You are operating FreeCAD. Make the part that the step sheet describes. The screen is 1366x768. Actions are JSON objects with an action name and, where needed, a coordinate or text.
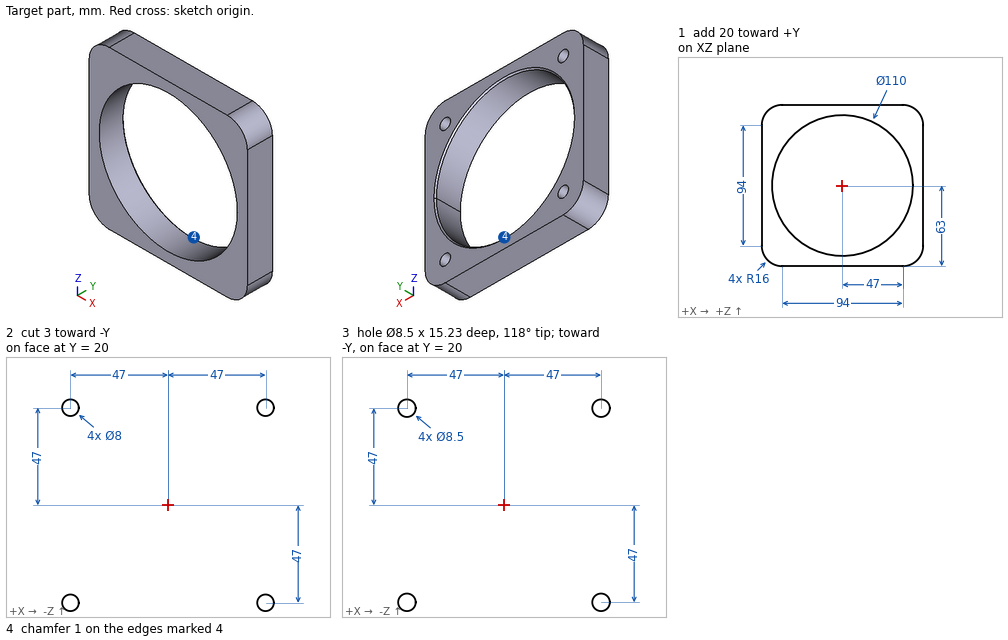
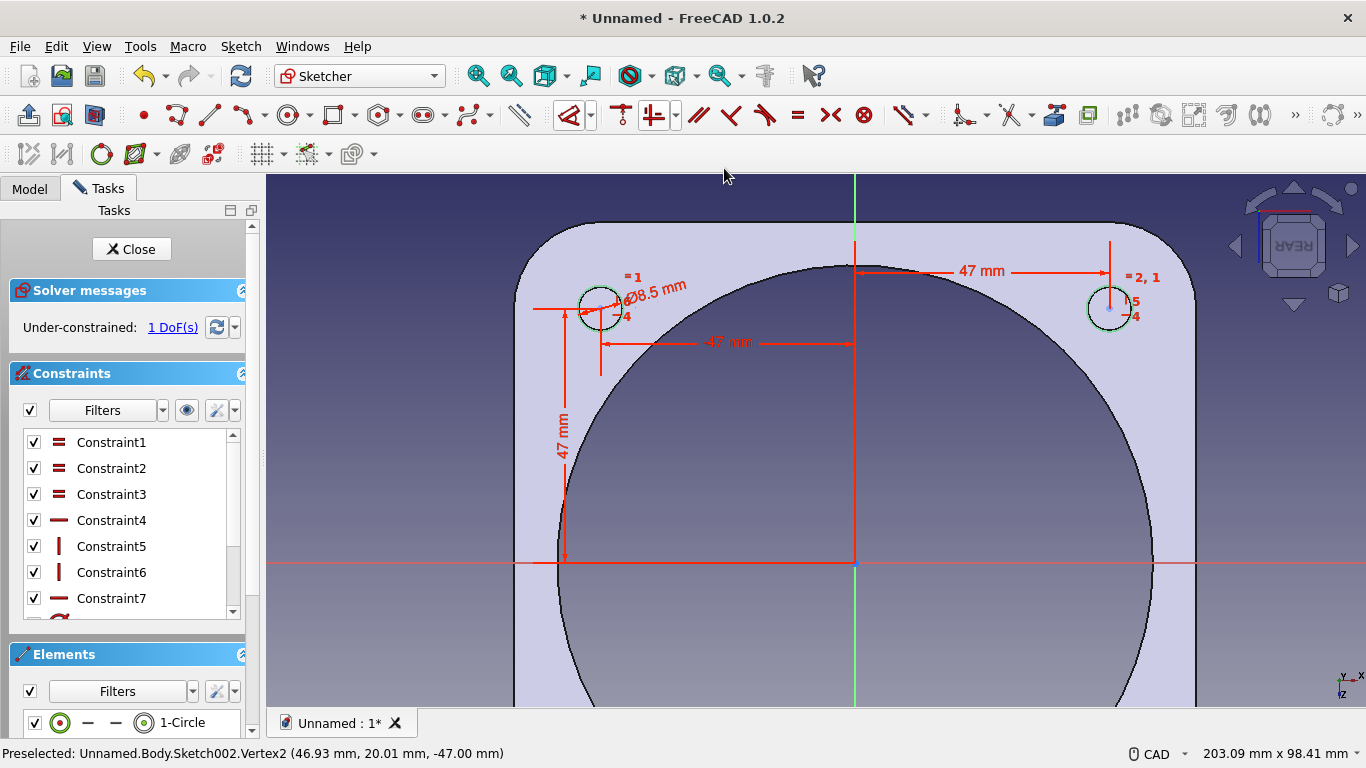
{"action": "scroll", "coordinate": [617, 291], "scroll_direction": "down", "scroll_amount": 3}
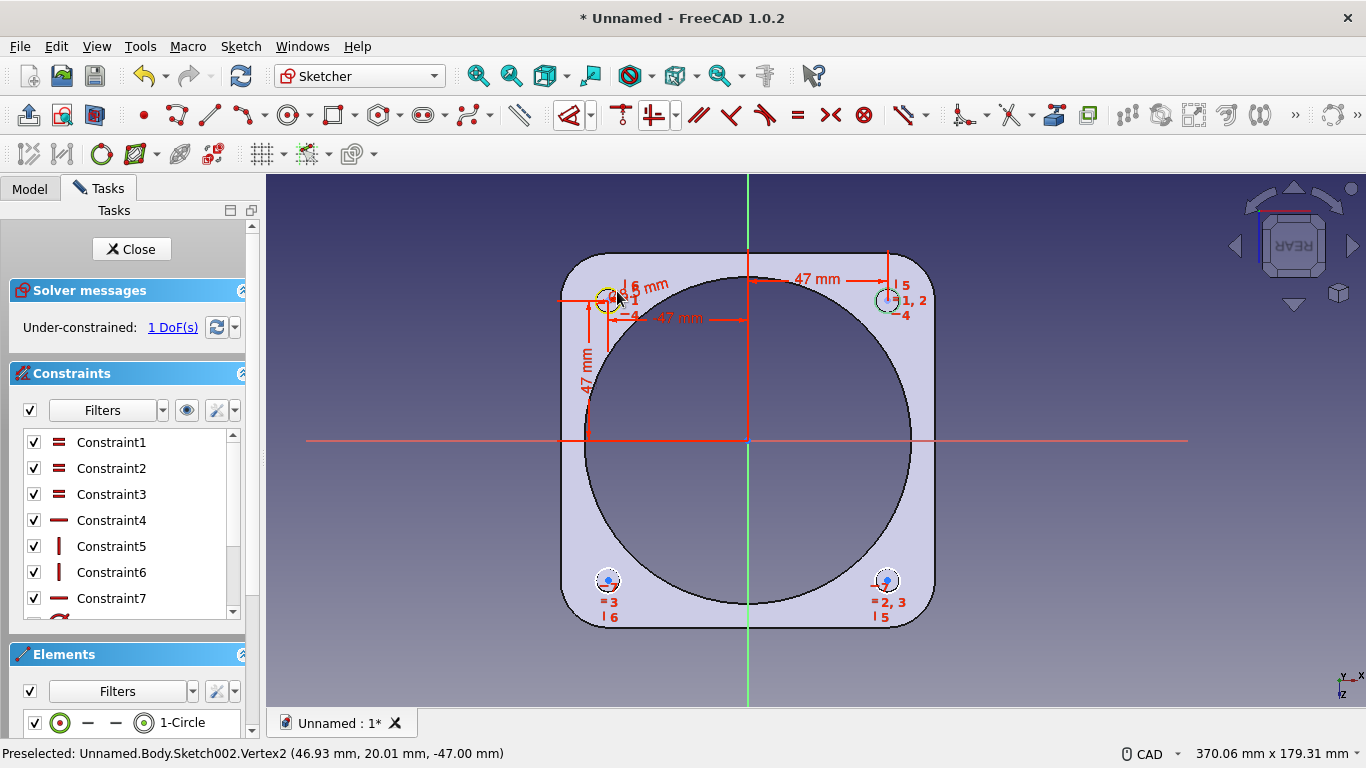
{"action": "left_click", "coordinate": [888, 581]}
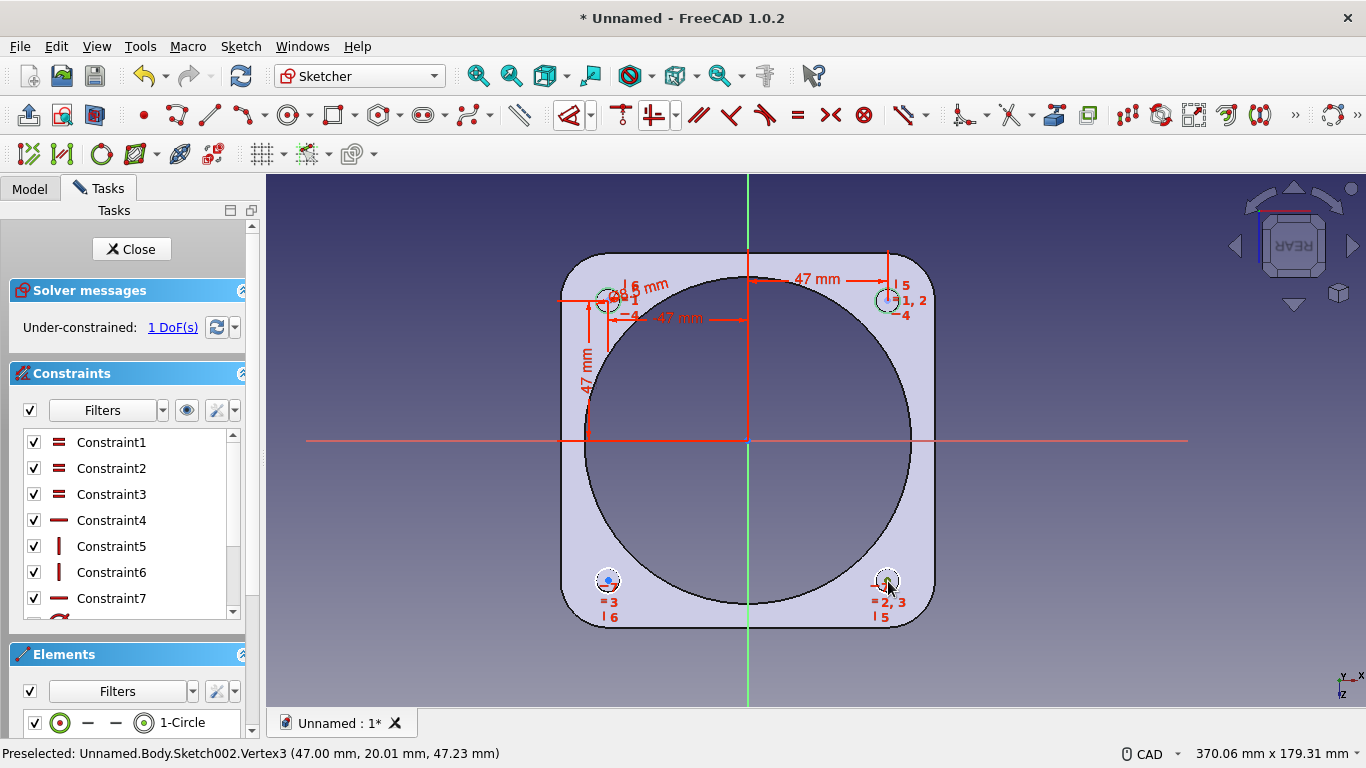
{"action": "left_click", "coordinate": [590, 116]}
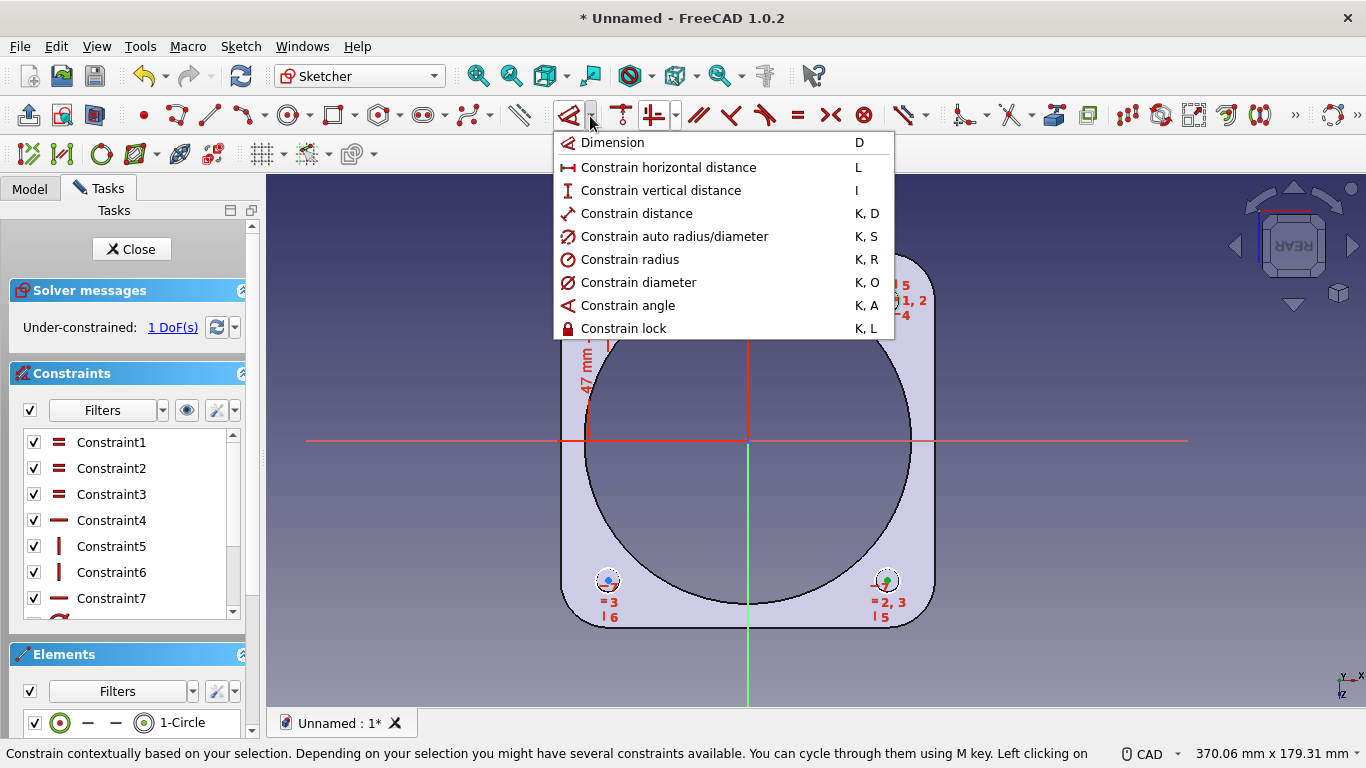
{"action": "left_click", "coordinate": [724, 190]}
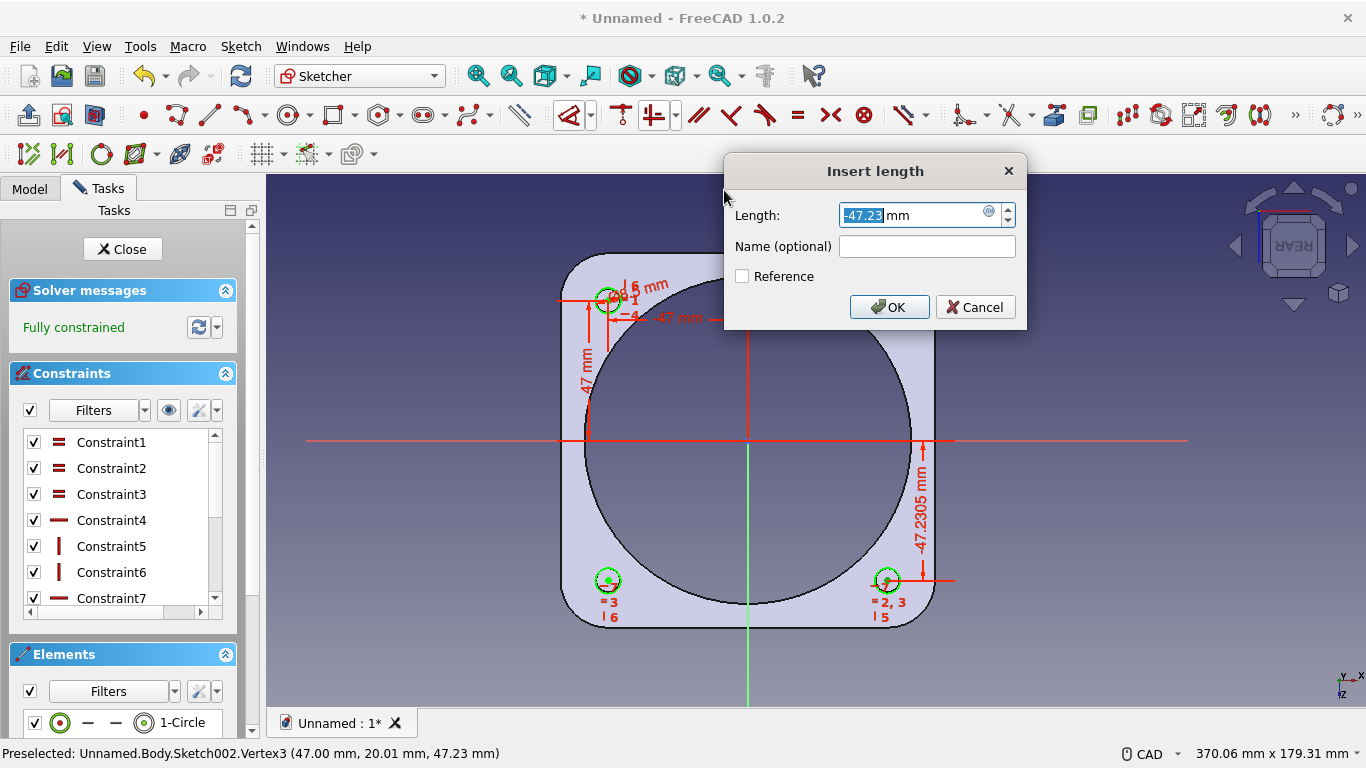
{"action": "type", "text": "-47"}
{"action": "key", "text": "Return"}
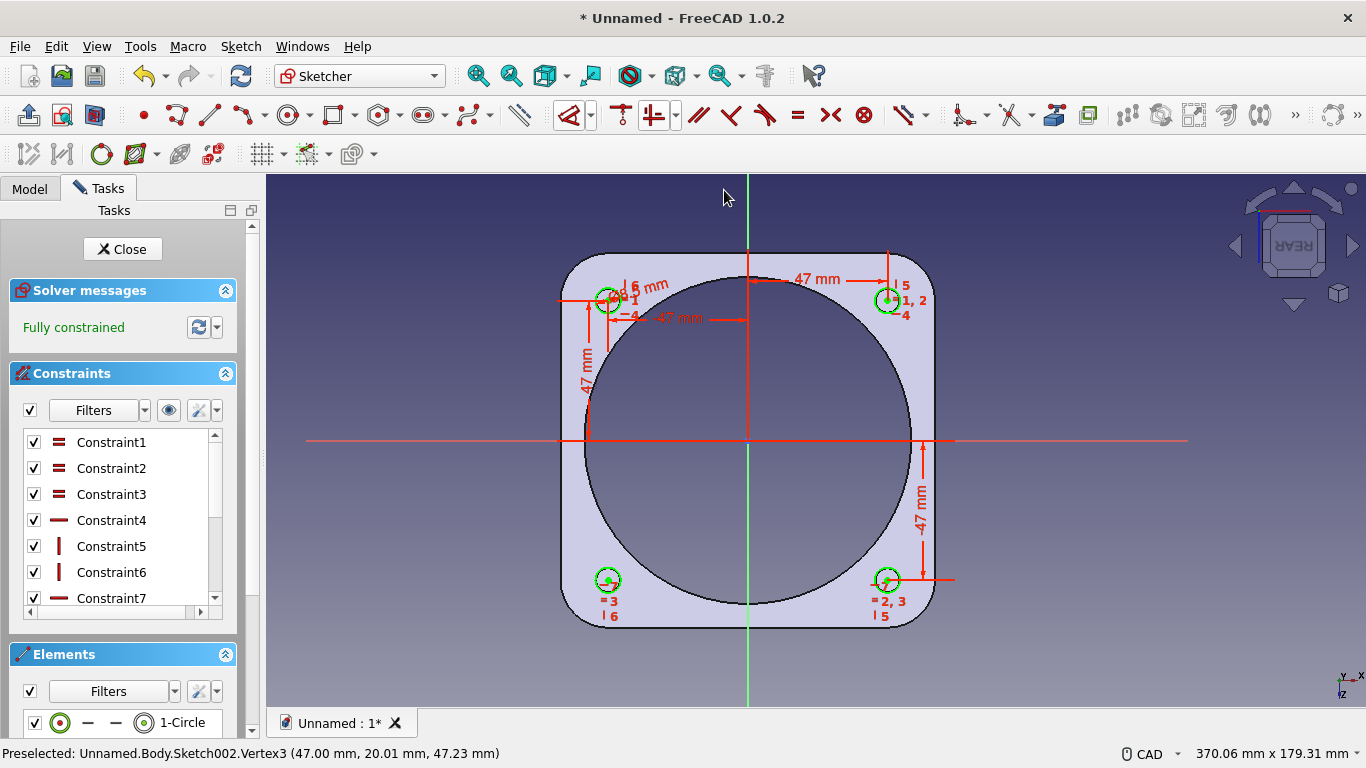
{"action": "left_click", "coordinate": [123, 249]}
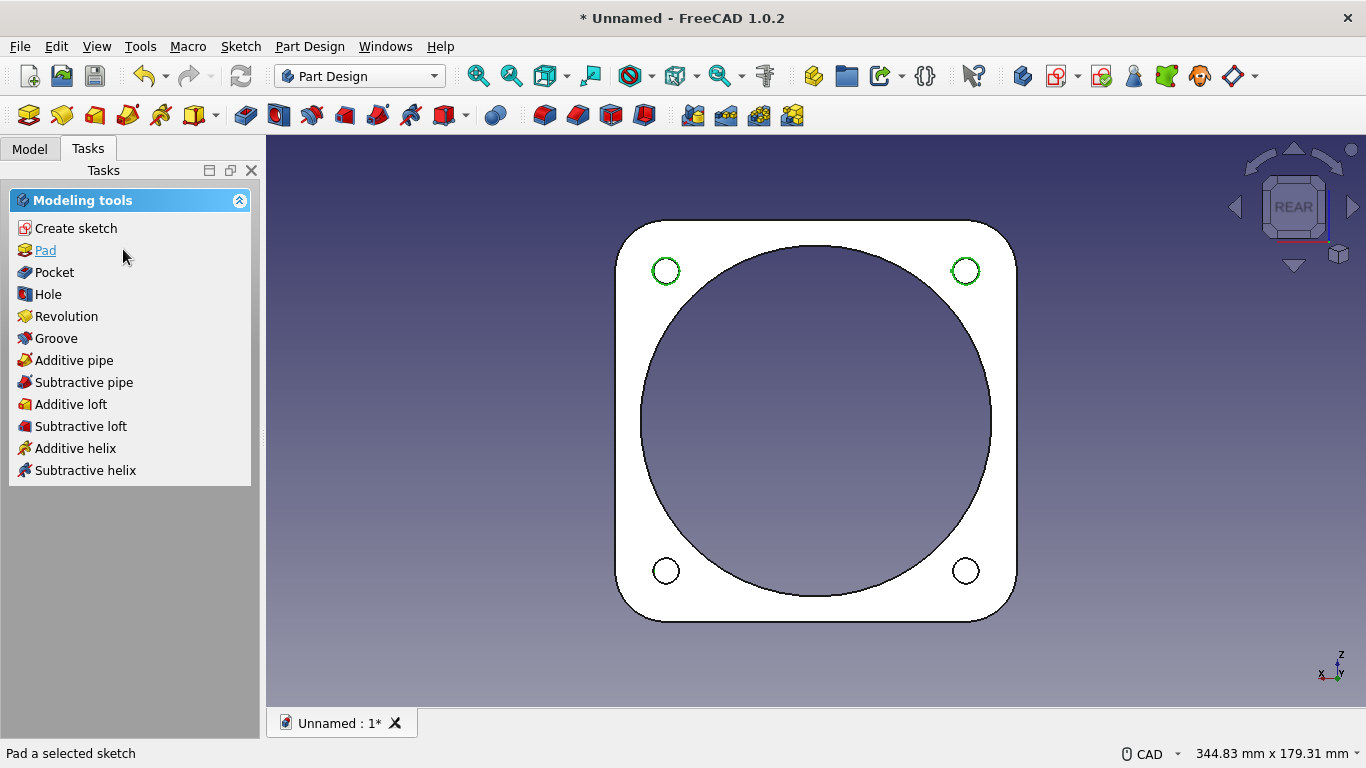
{"action": "left_click", "coordinate": [279, 116]}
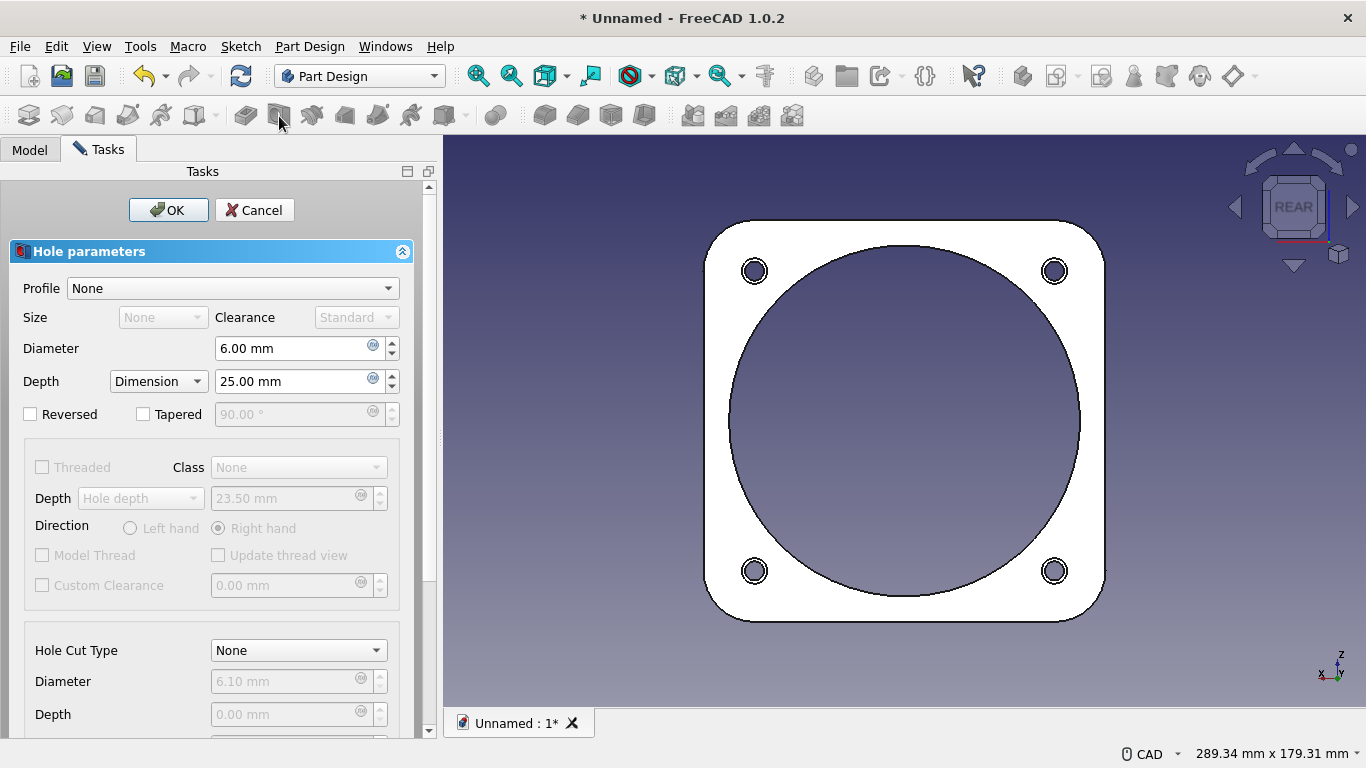
{"action": "triple_click", "coordinate": [300, 348]}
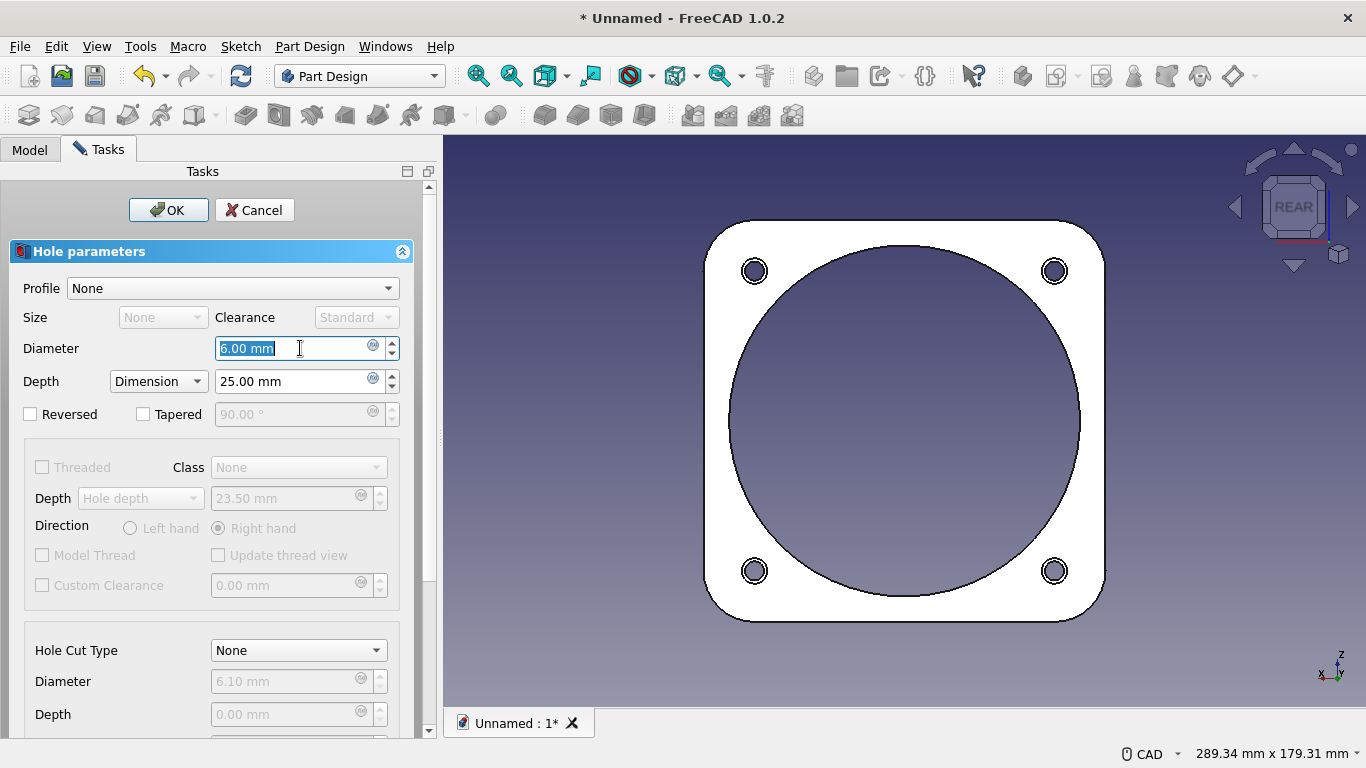
{"action": "type", "text": "8.5"}
{"action": "key", "text": "Tab"}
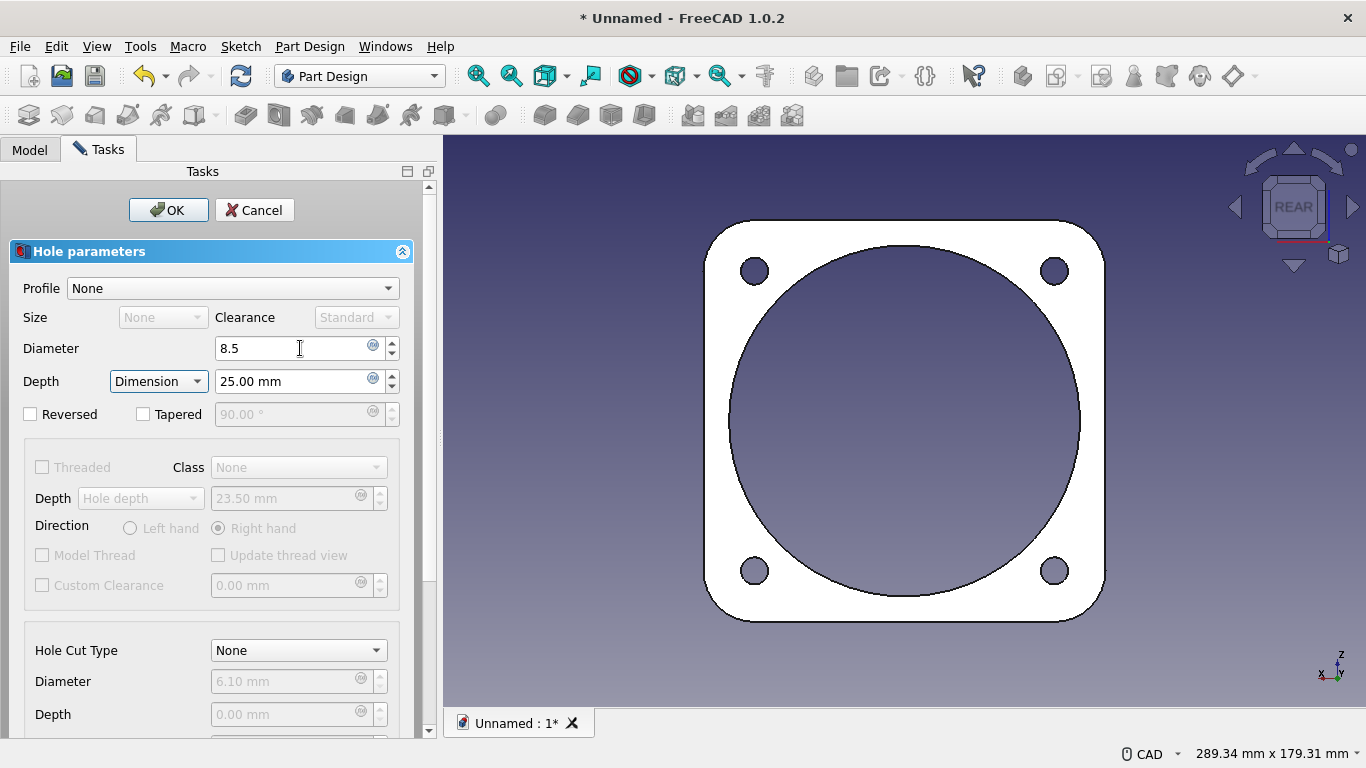
{"action": "triple_click", "coordinate": [300, 382]}